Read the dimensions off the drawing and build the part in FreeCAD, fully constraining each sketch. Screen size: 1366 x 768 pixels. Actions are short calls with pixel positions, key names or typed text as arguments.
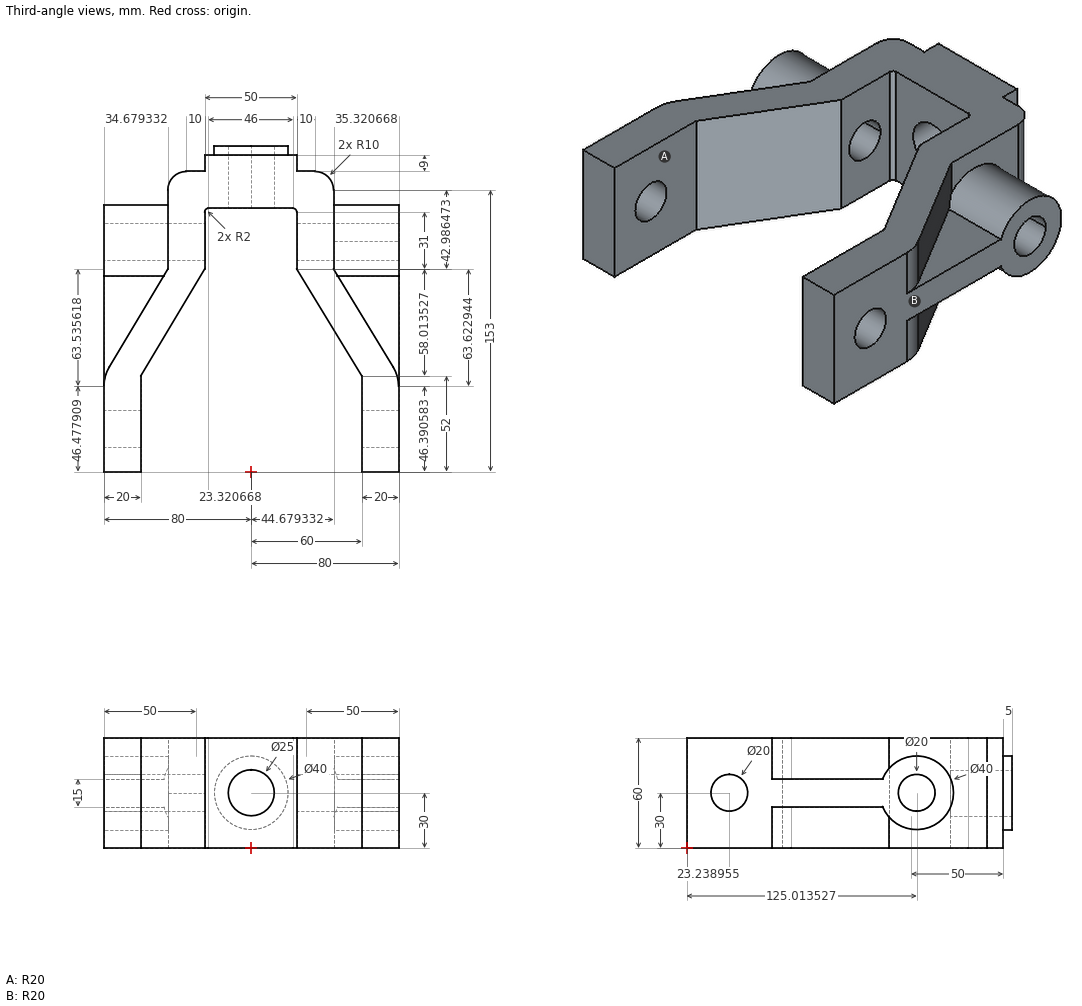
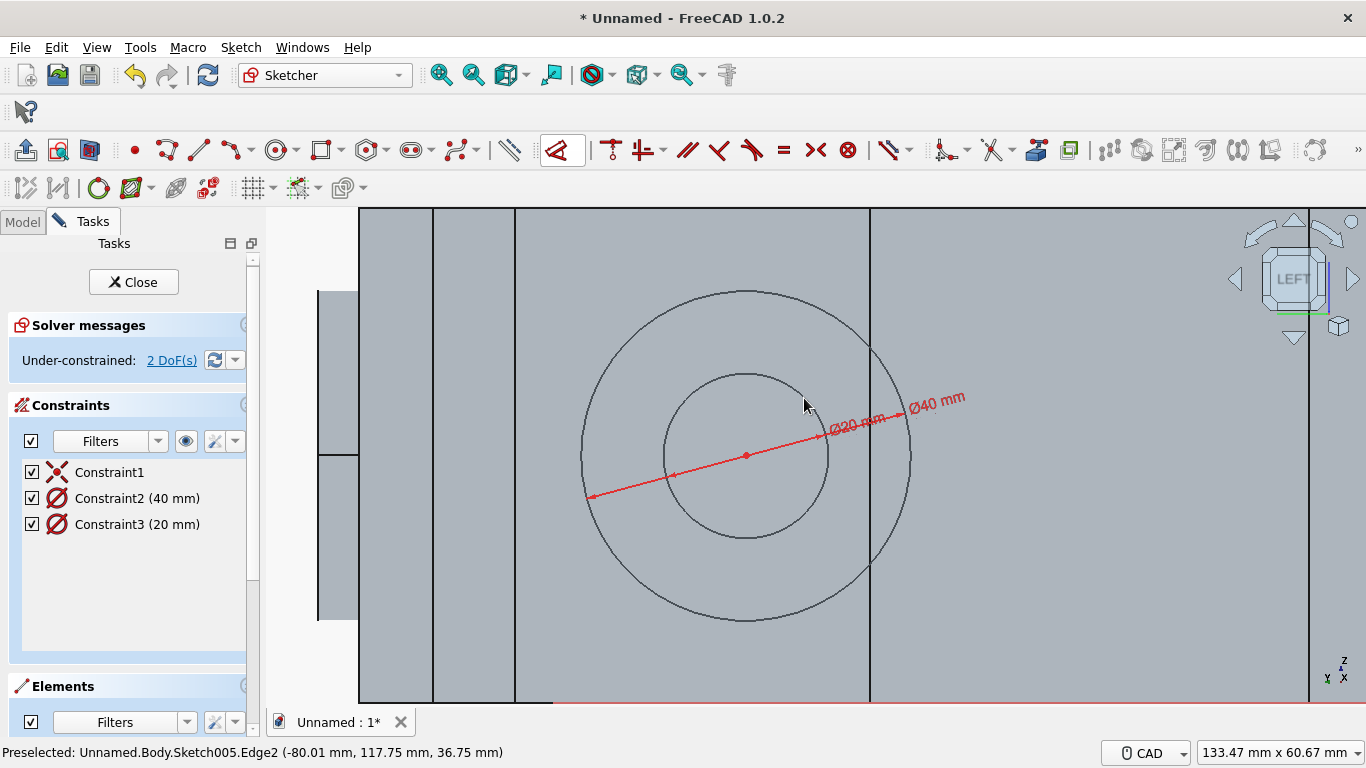
click(746, 456)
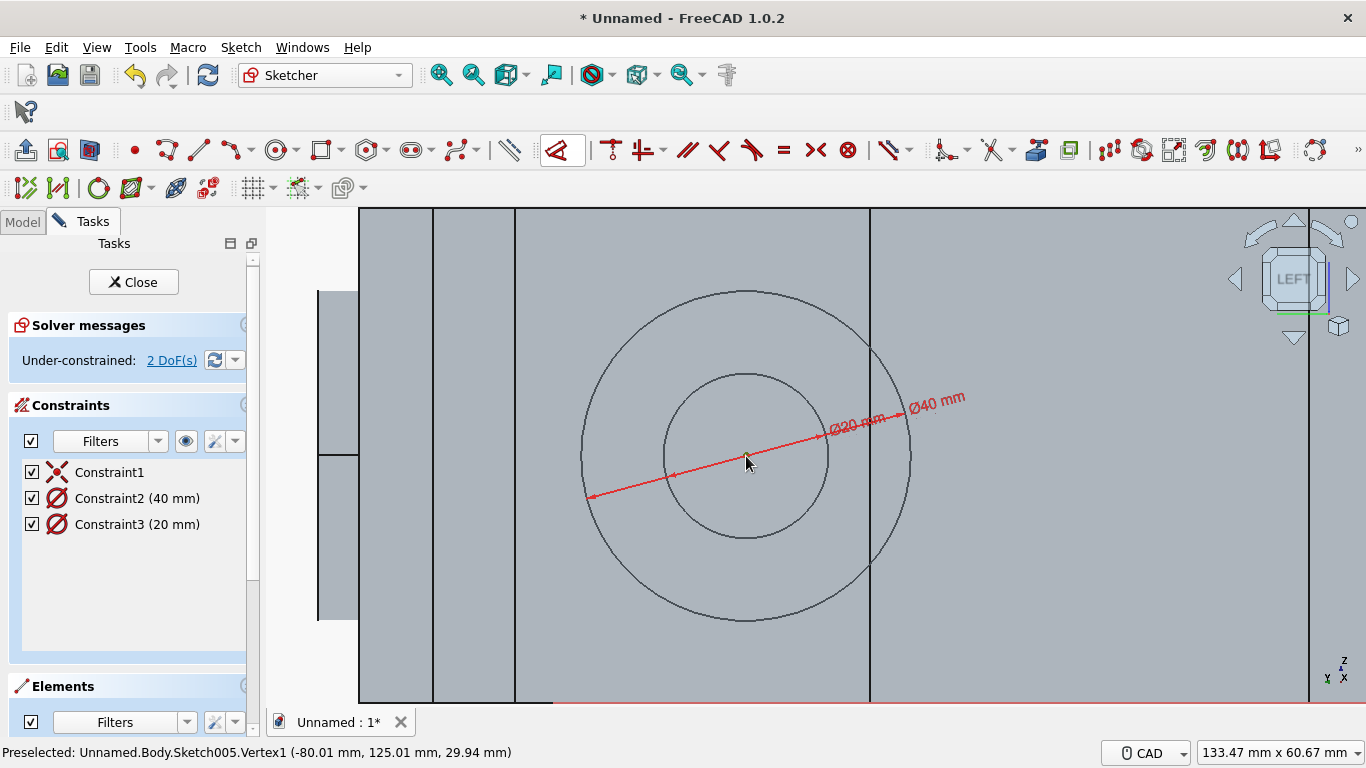
key(i)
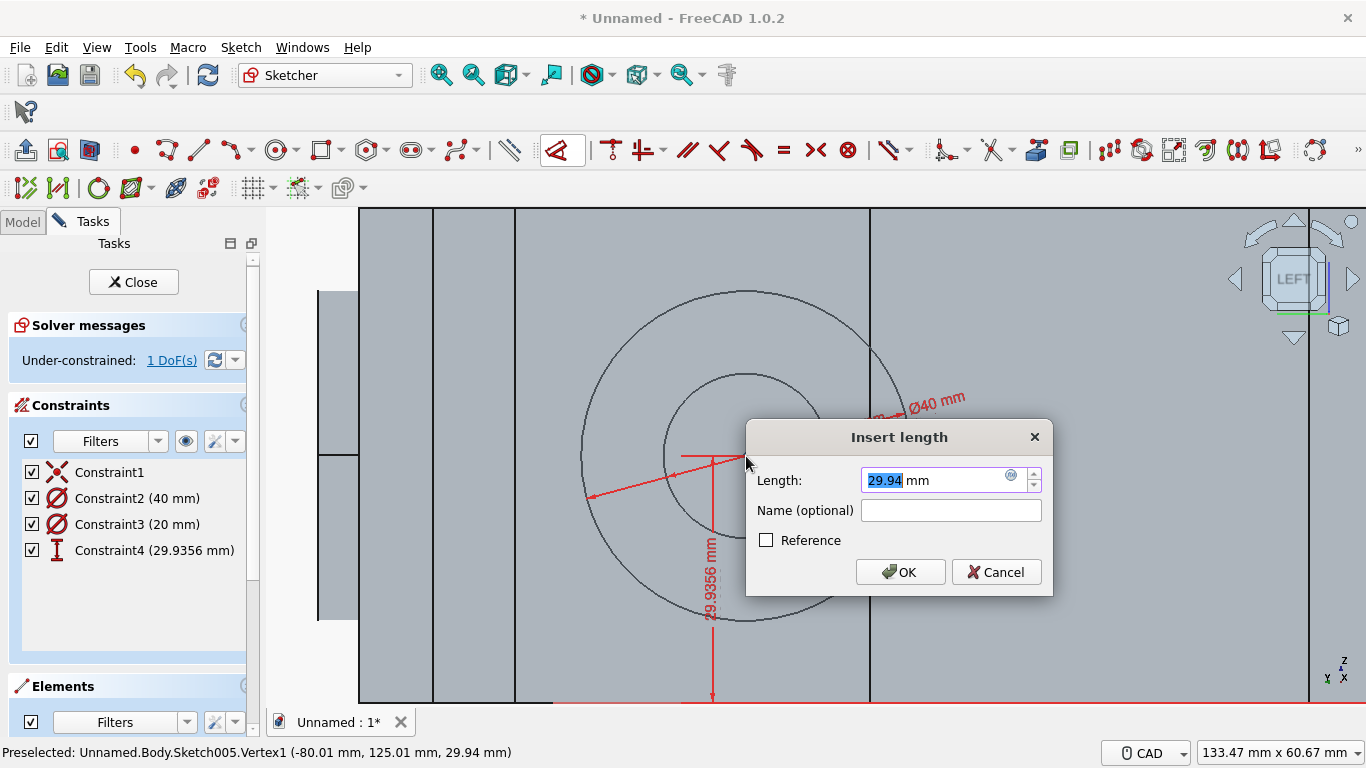
text(30)
key(Return)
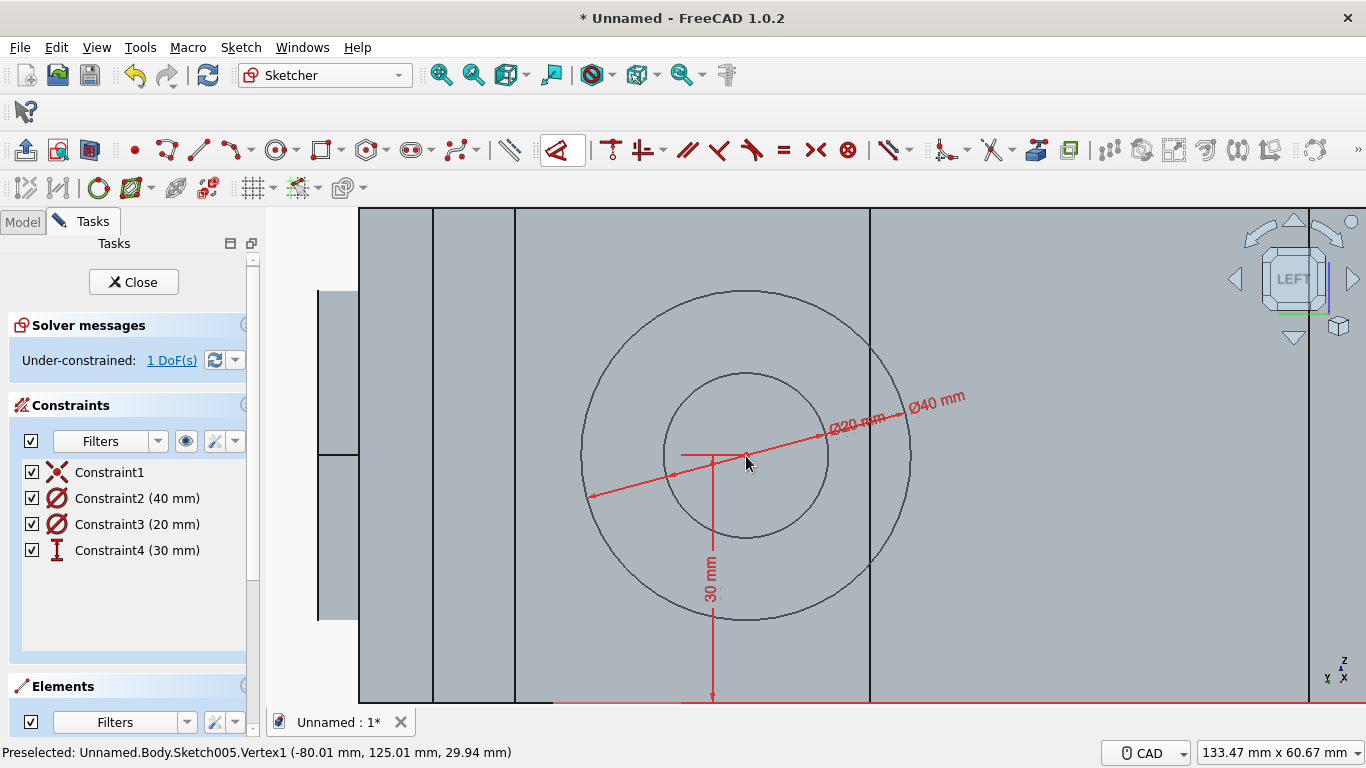
click(746, 455)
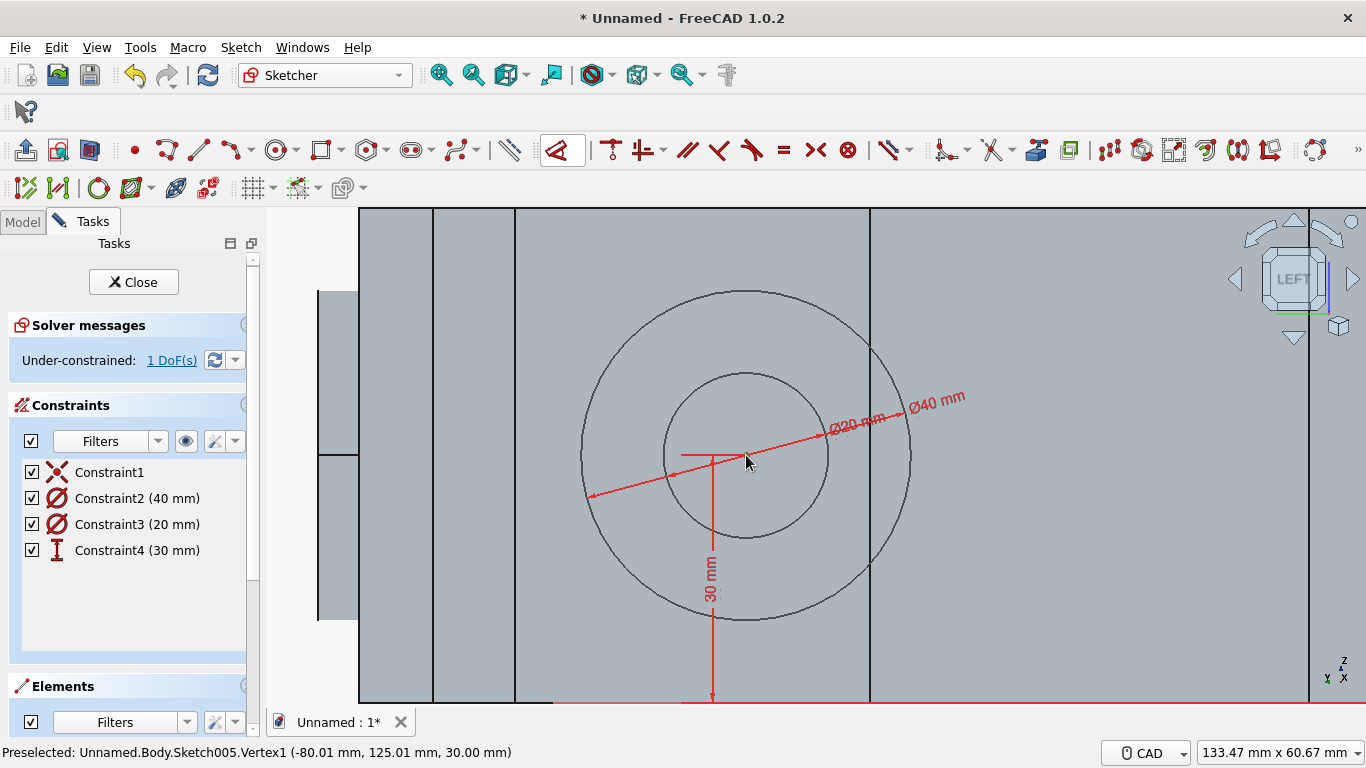
click(580, 150)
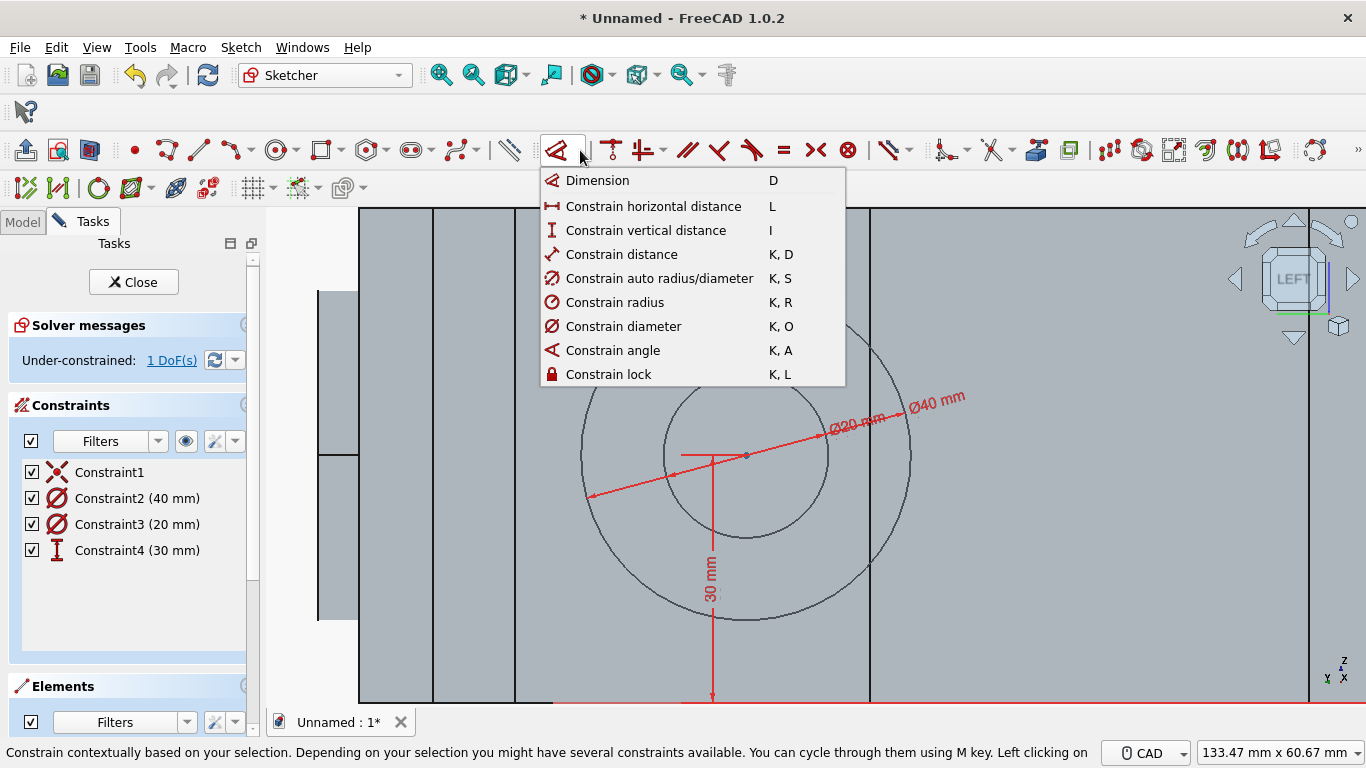
click(693, 206)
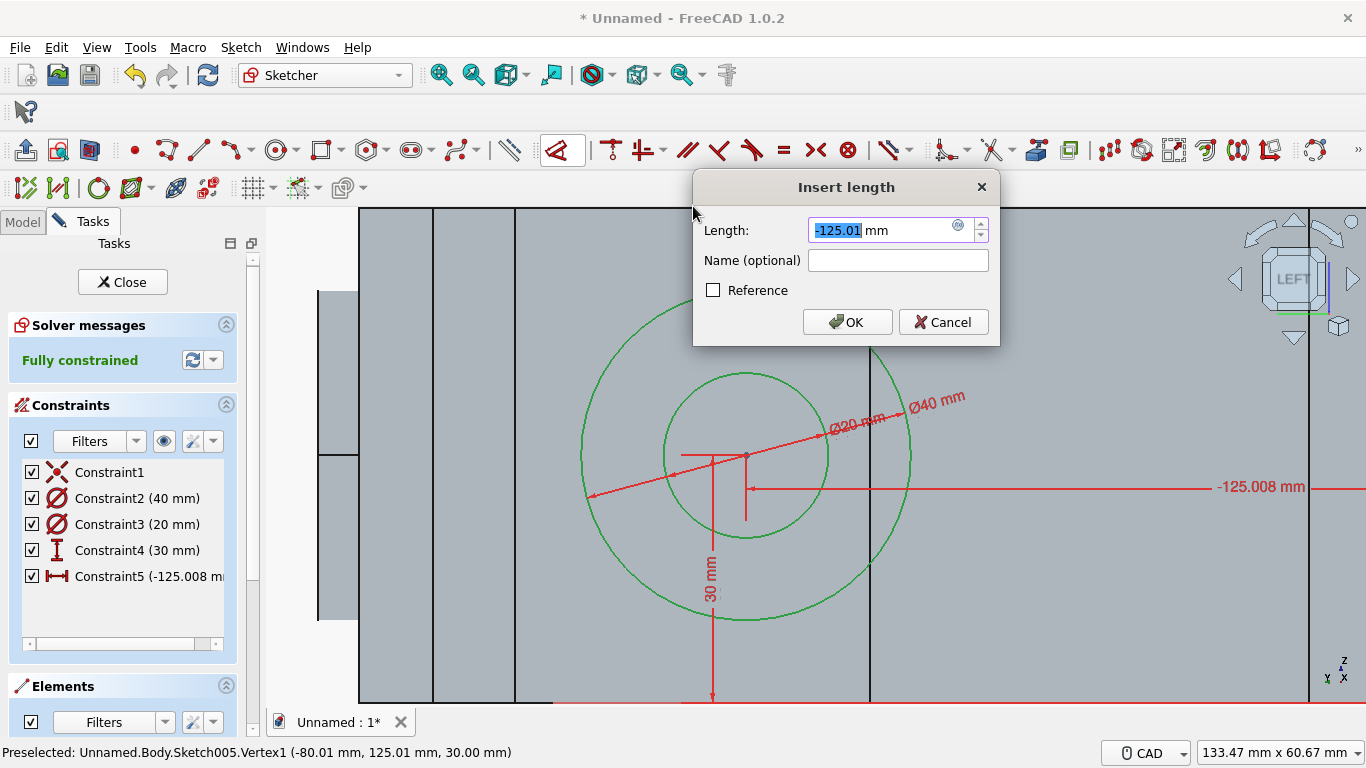
text(-125.013527)
key(Return)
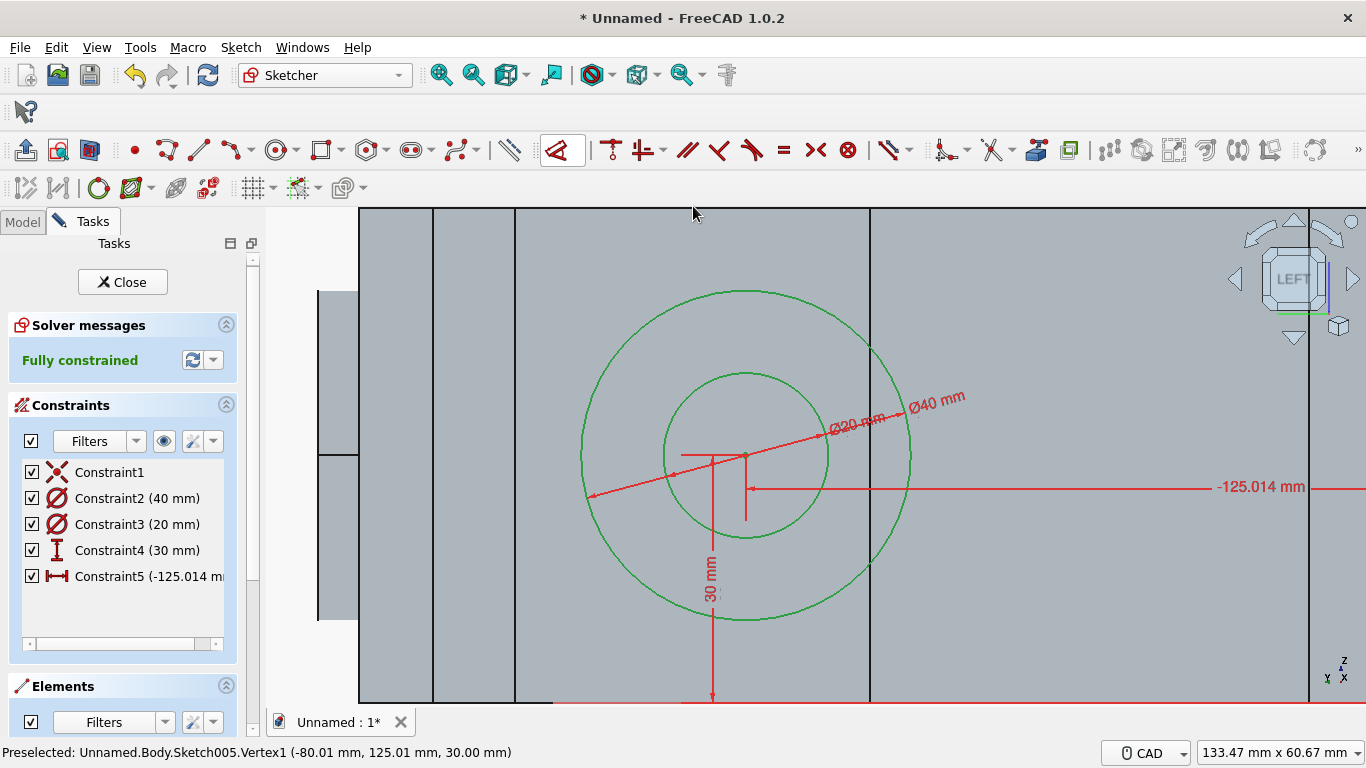
click(123, 282)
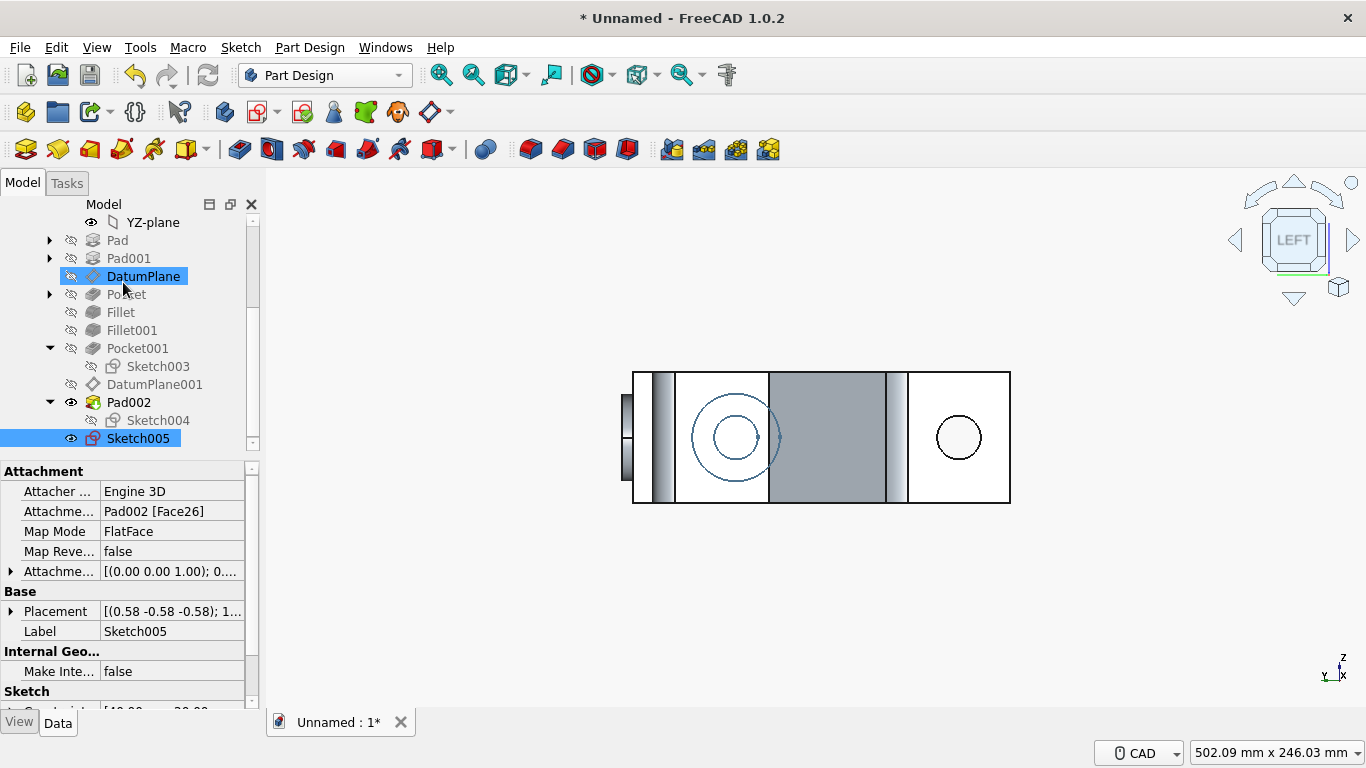
click(26, 150)